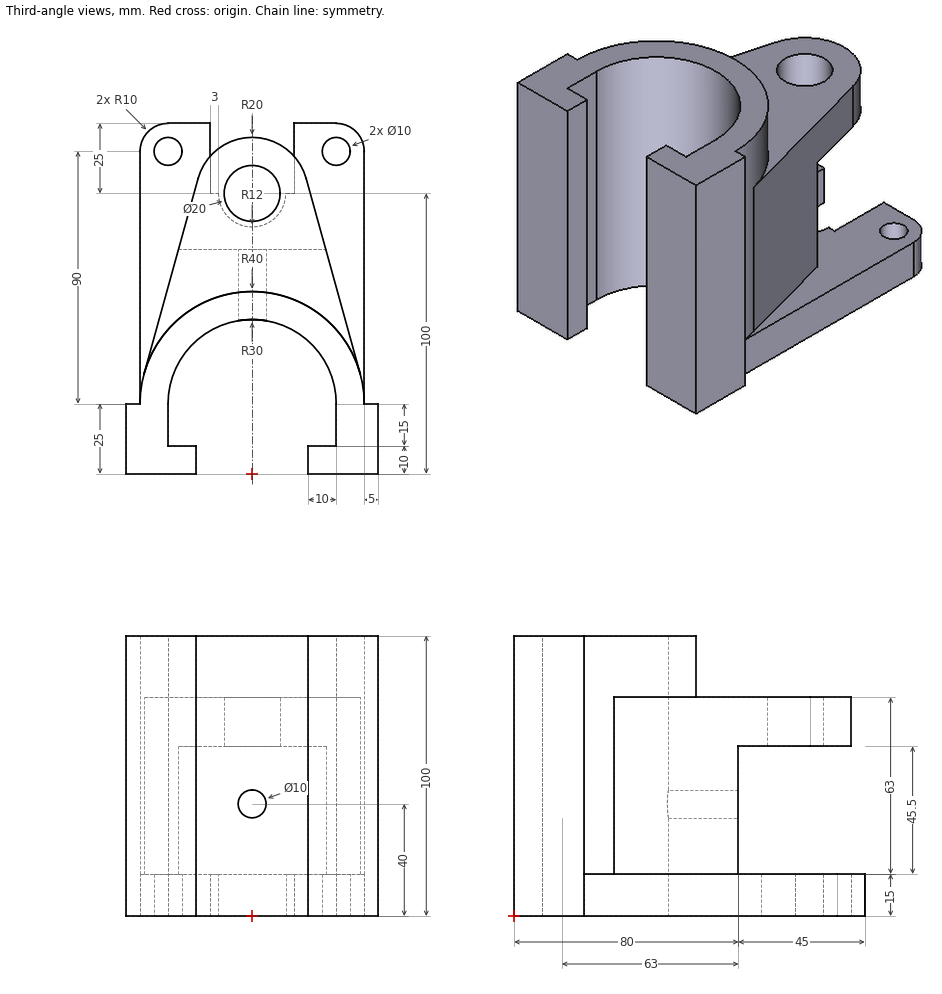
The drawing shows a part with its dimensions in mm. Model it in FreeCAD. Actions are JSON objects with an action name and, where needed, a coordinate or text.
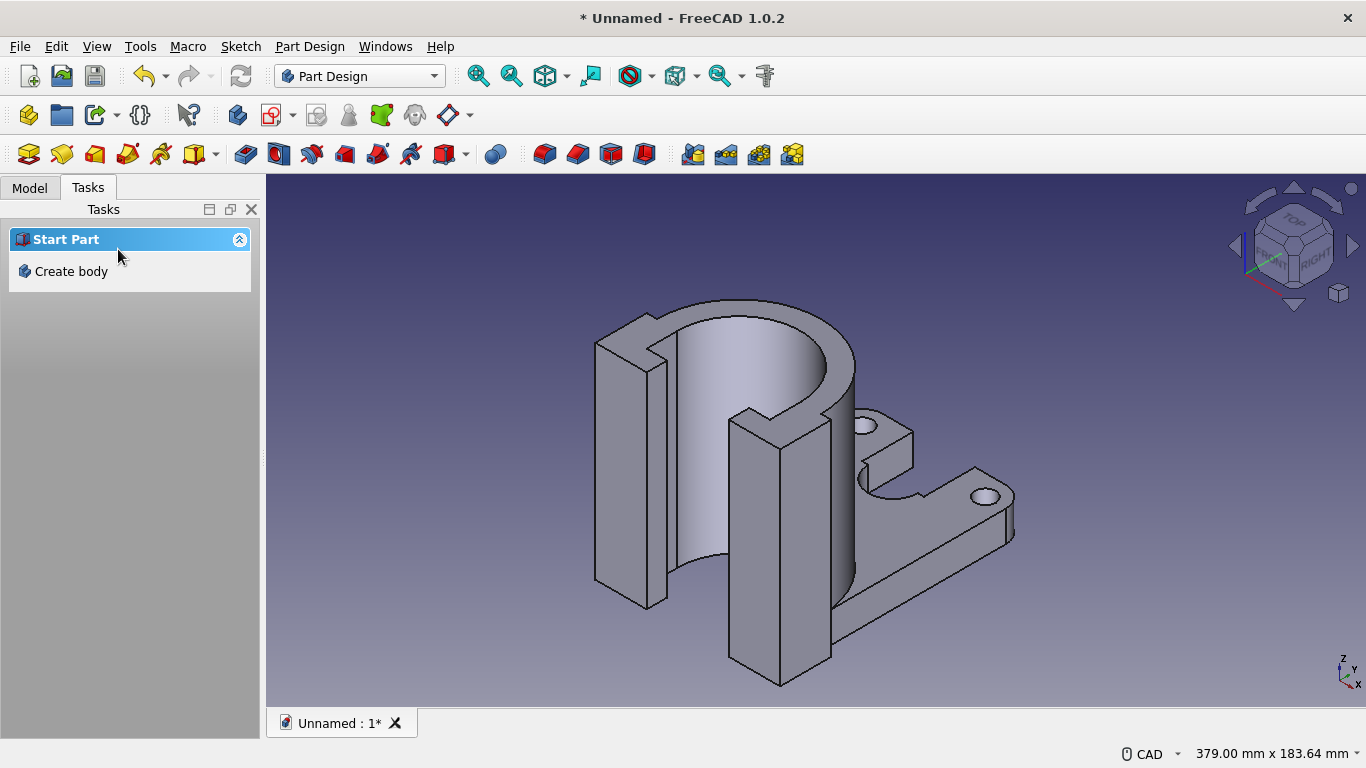
{"action": "left_click", "coordinate": [889, 535]}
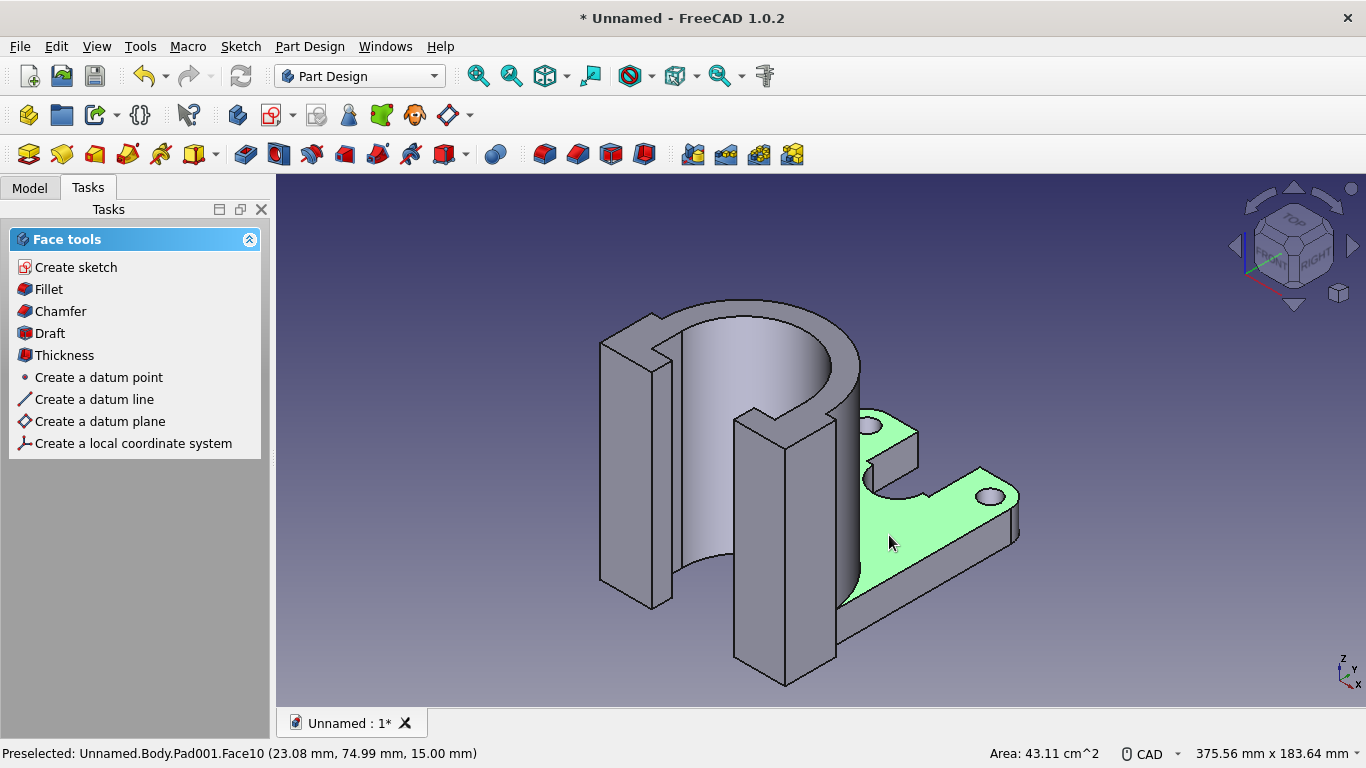
{"action": "left_click", "coordinate": [270, 116]}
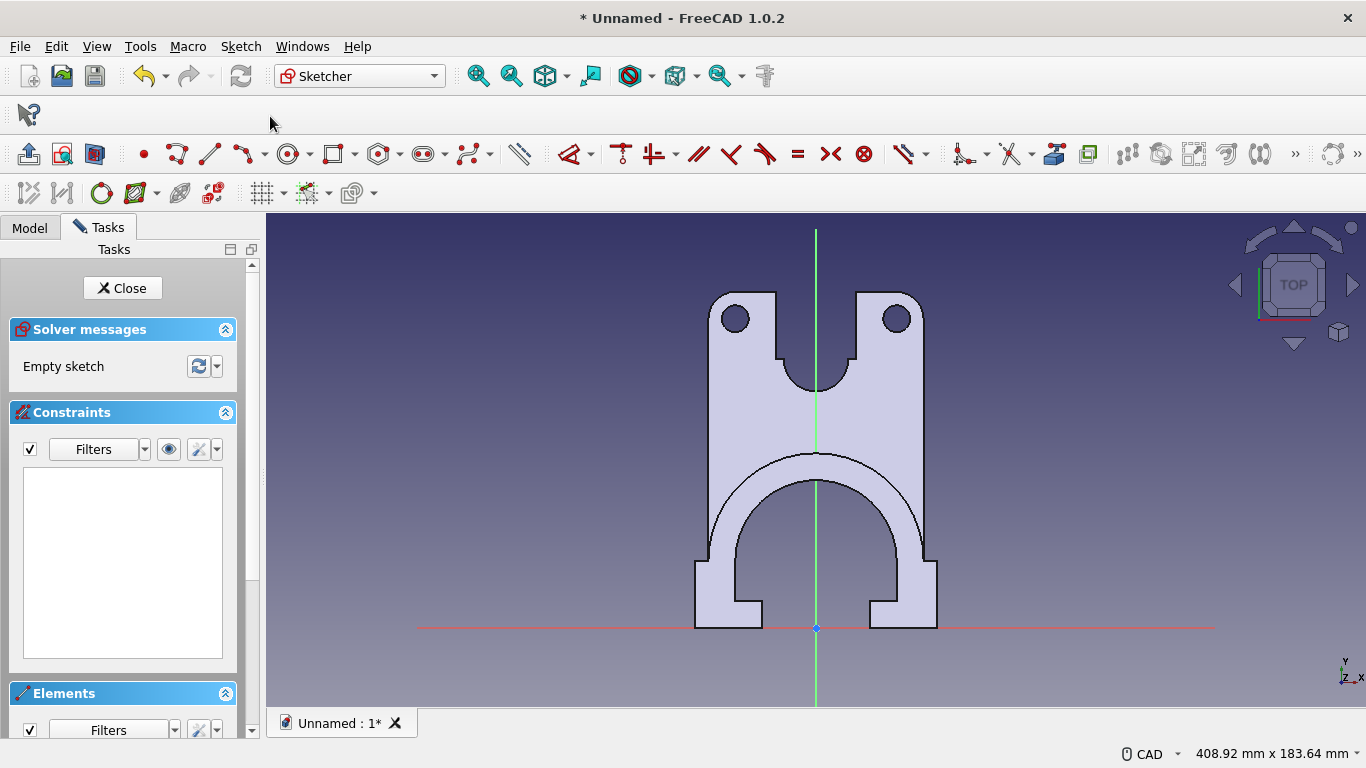
{"action": "key", "text": "g l"}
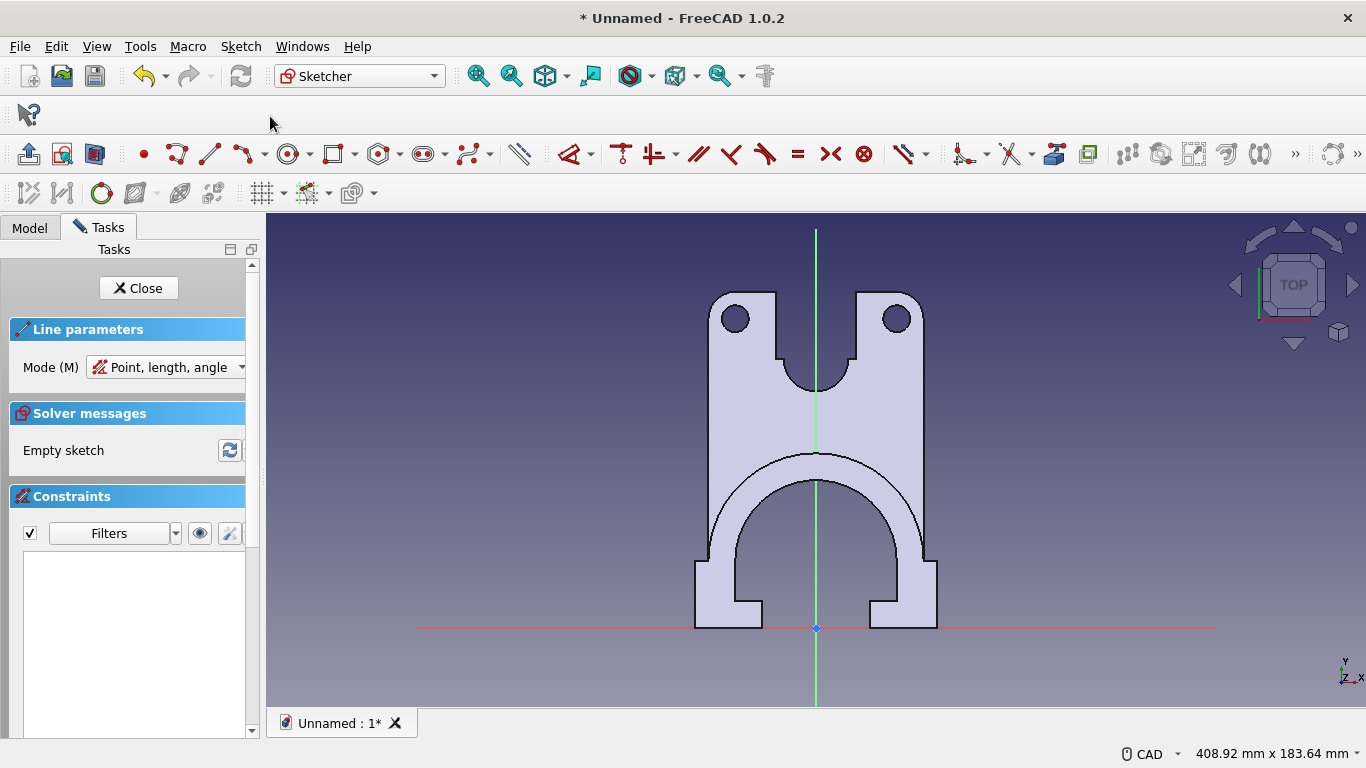
{"action": "left_click", "coordinate": [764, 345]}
{"action": "left_click", "coordinate": [712, 532]}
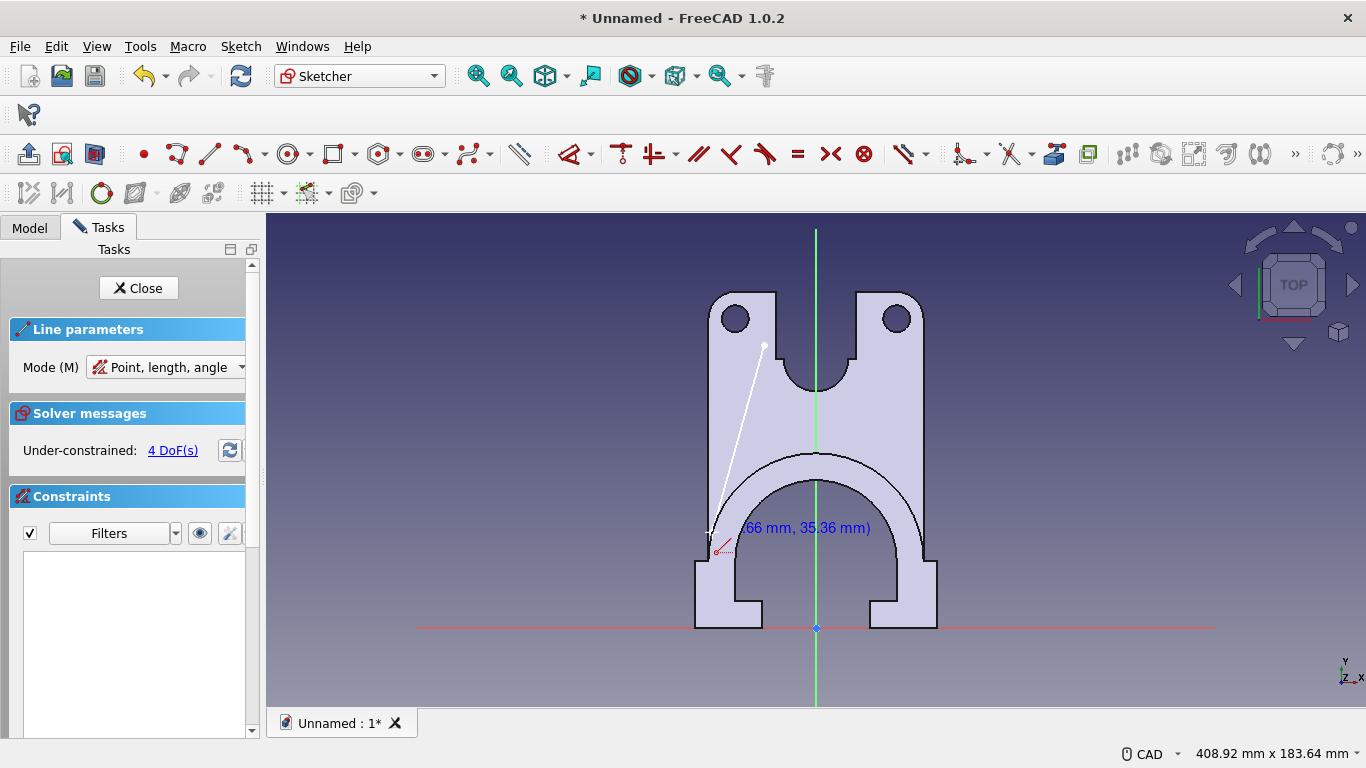
{"action": "left_click", "coordinate": [920, 532]}
{"action": "left_click", "coordinate": [868, 345]}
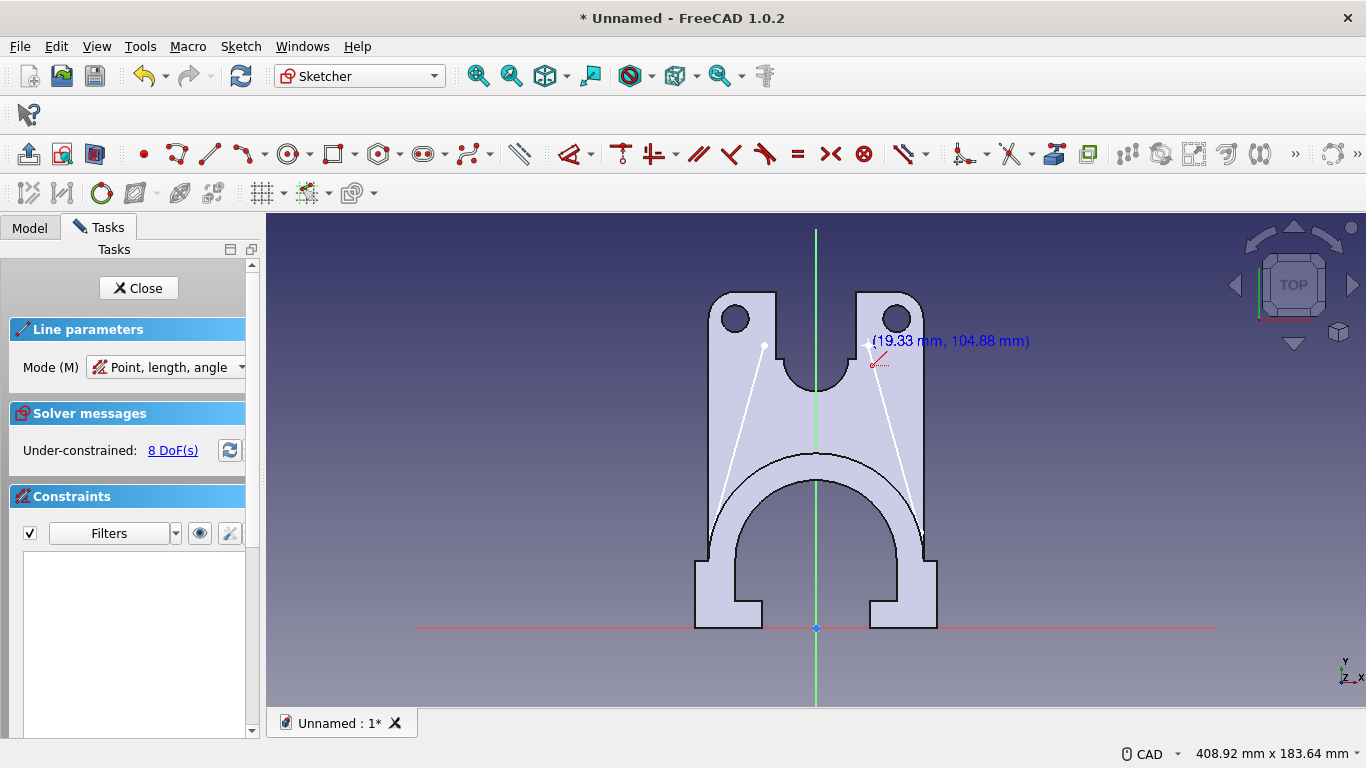
{"action": "key", "text": "g 3 a"}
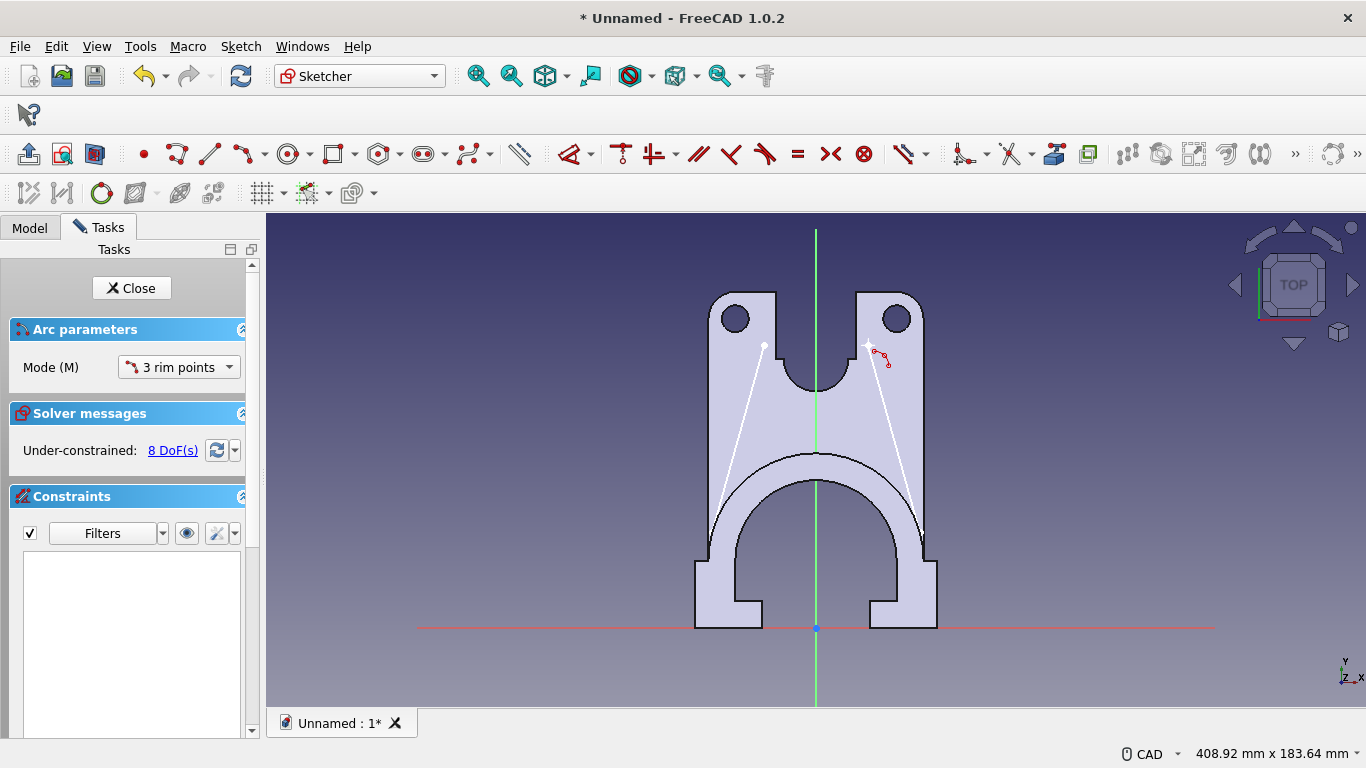
{"action": "left_click", "coordinate": [712, 533]}
{"action": "left_click", "coordinate": [920, 533]}
{"action": "left_click", "coordinate": [844, 457]}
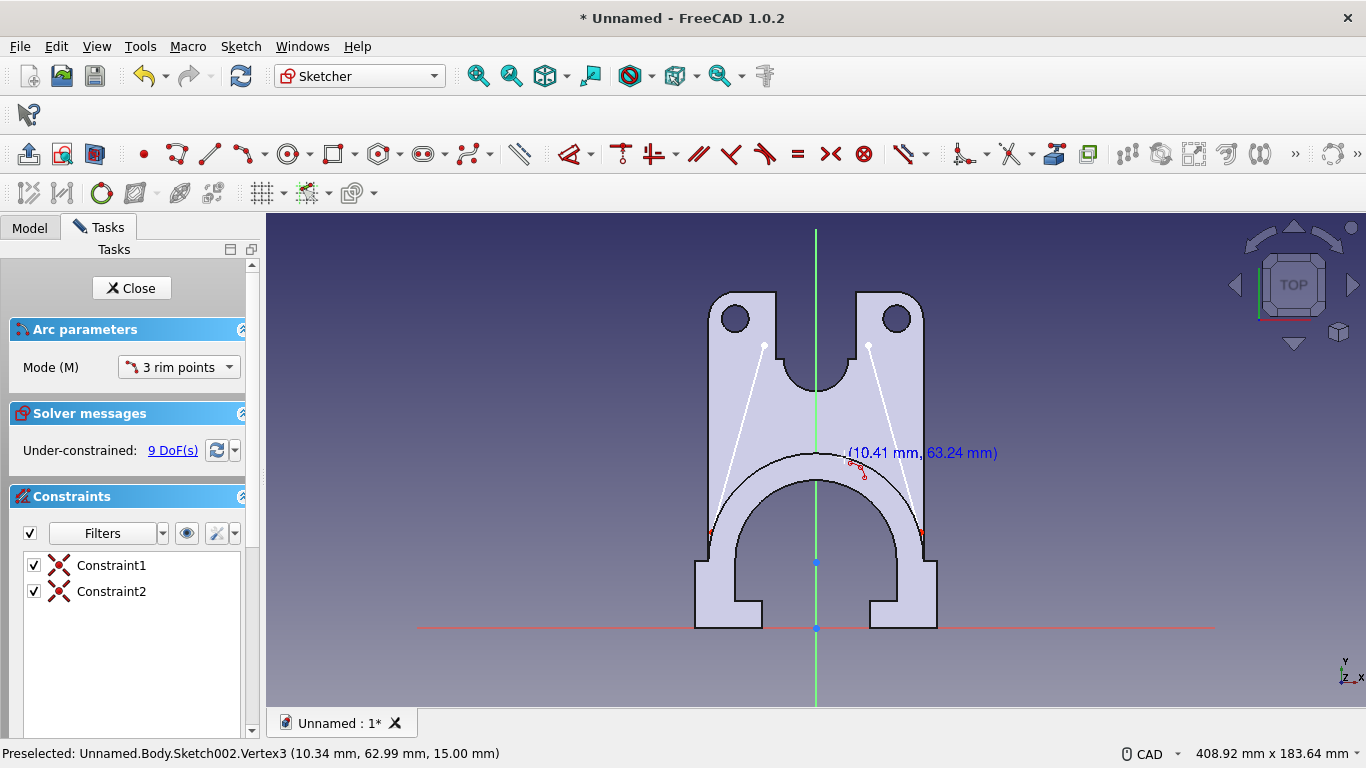
{"action": "left_click", "coordinate": [868, 346]}
{"action": "left_click", "coordinate": [764, 346]}
{"action": "left_click", "coordinate": [843, 312]}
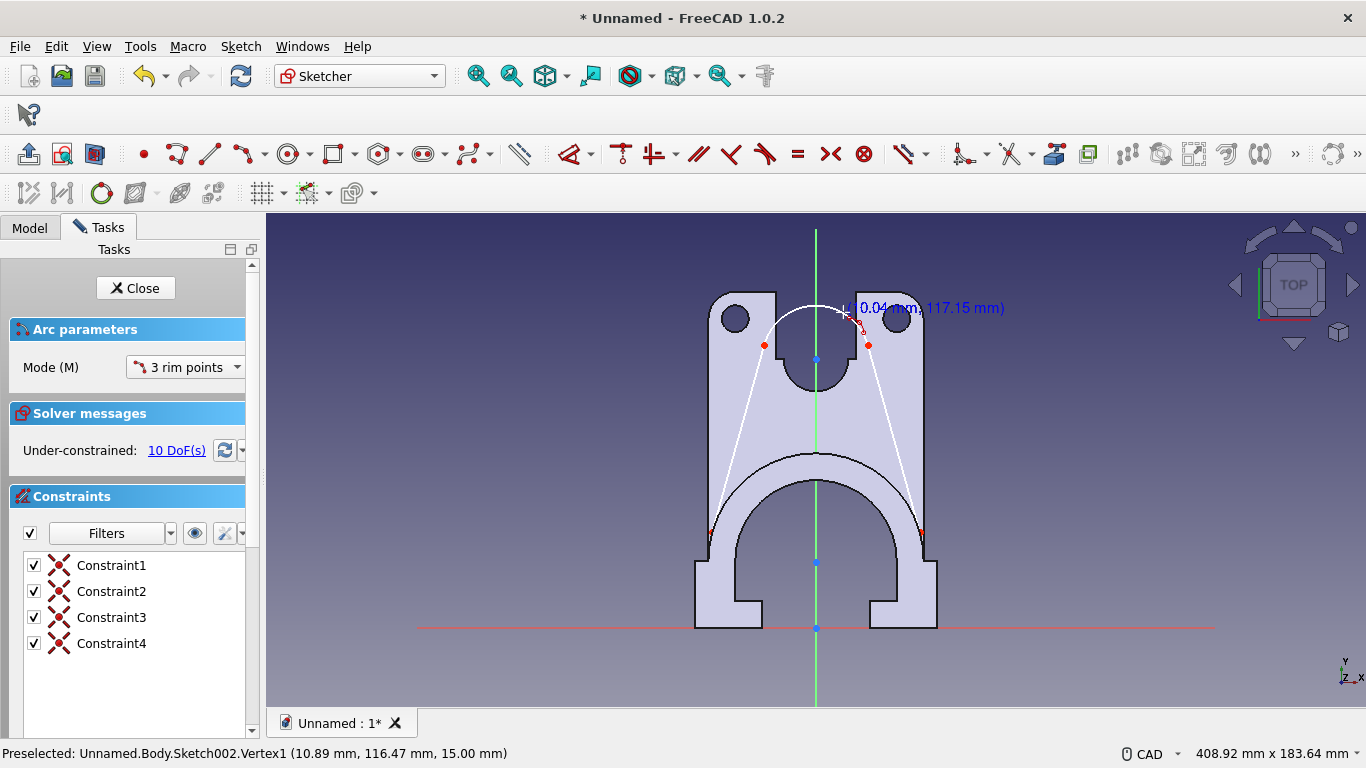
{"action": "key", "text": "g c"}